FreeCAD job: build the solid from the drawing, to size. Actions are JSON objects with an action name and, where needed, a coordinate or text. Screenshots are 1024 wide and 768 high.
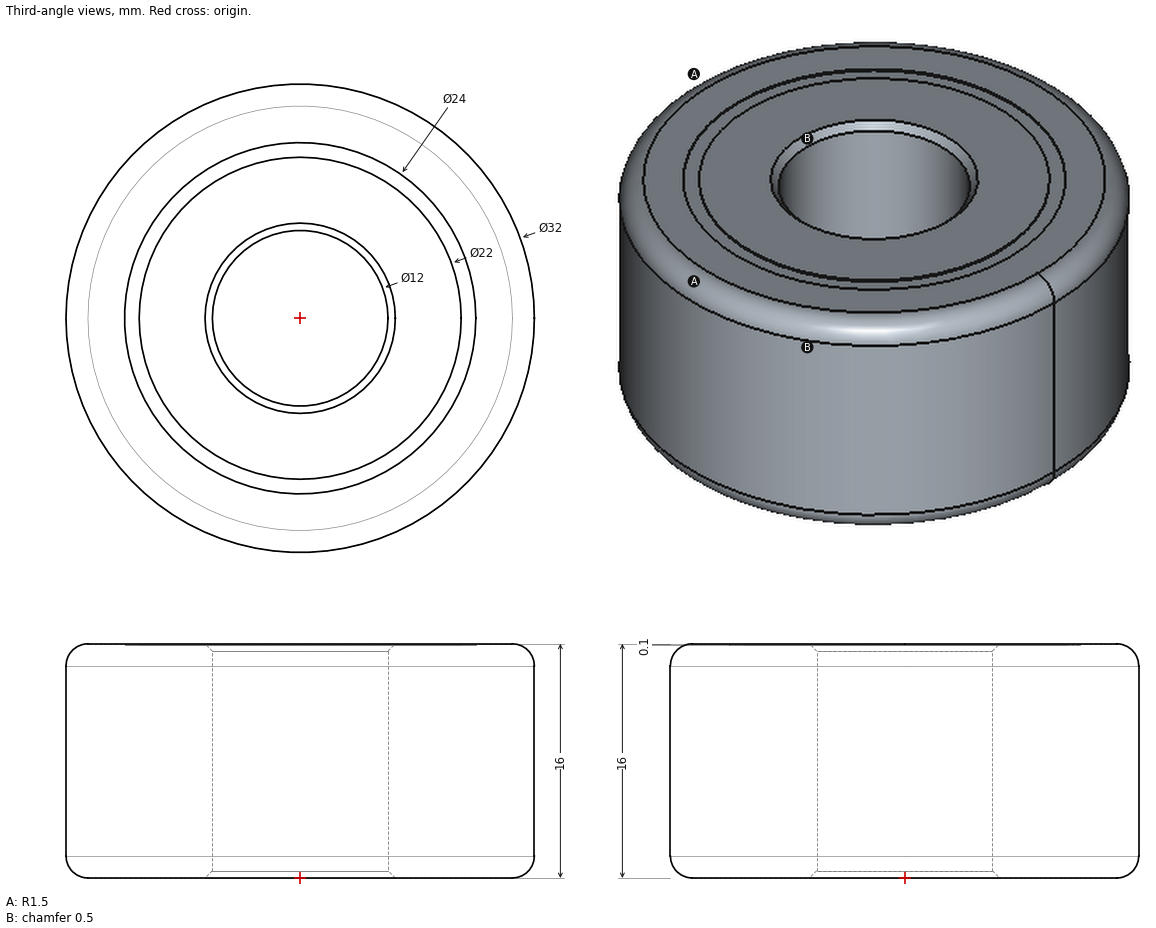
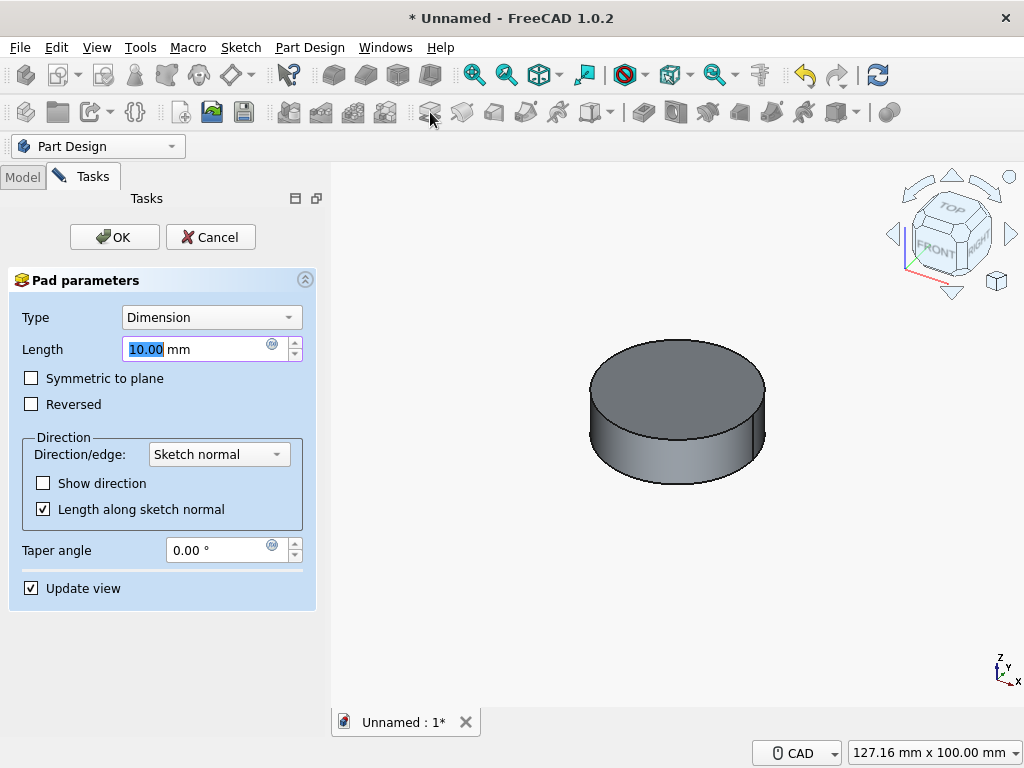
{"action": "type", "text": "16"}
{"action": "key", "text": "Tab"}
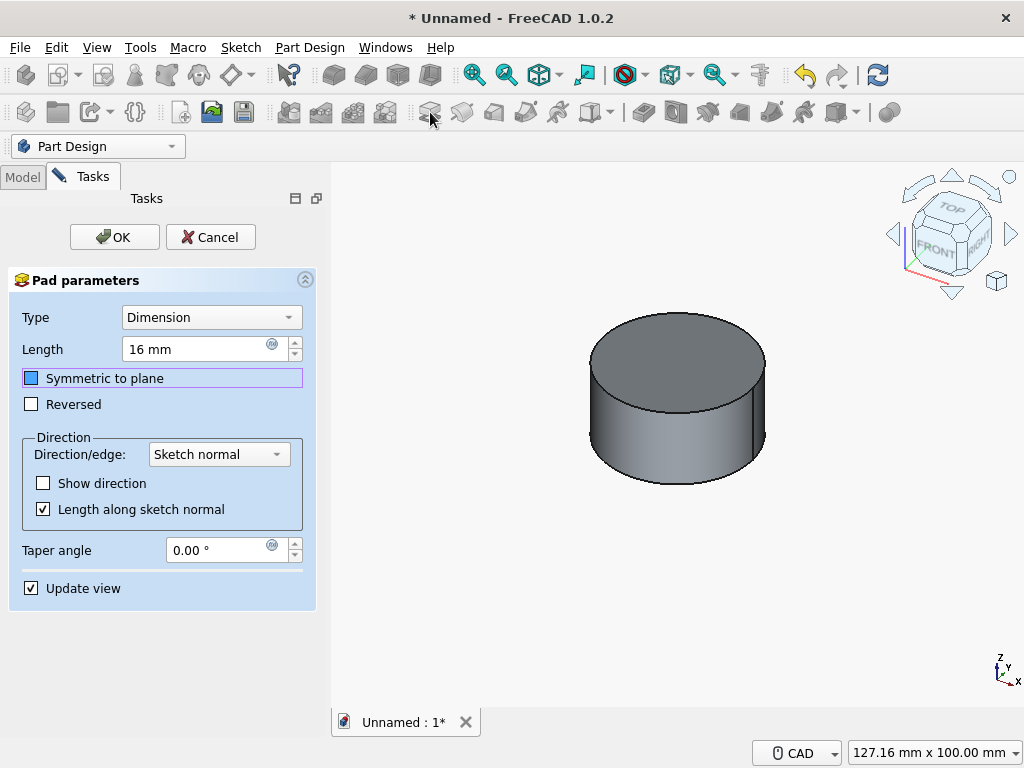
{"action": "left_click", "coordinate": [115, 237]}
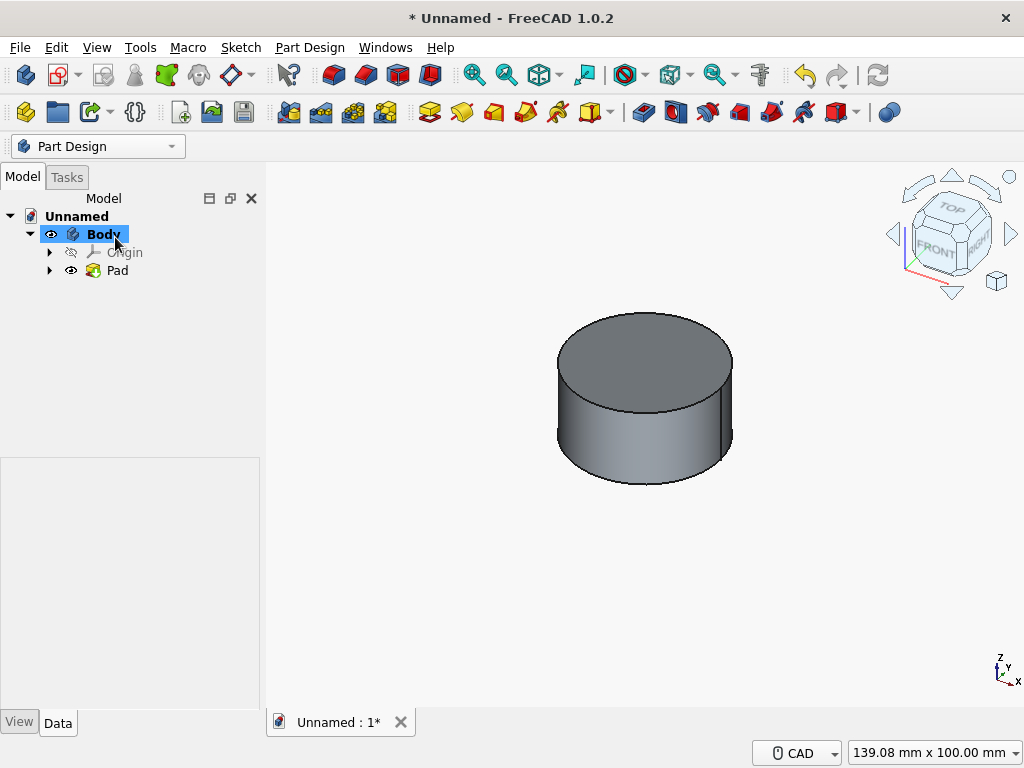
{"action": "left_click", "coordinate": [476, 76]}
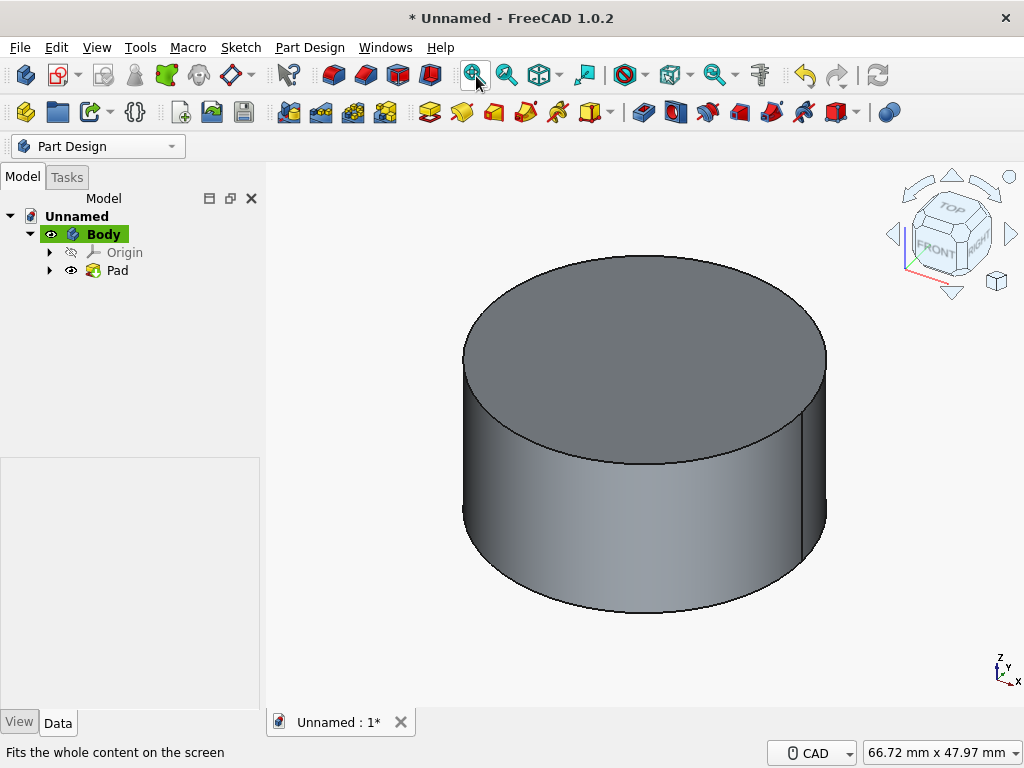
{"action": "left_click", "coordinate": [645, 359]}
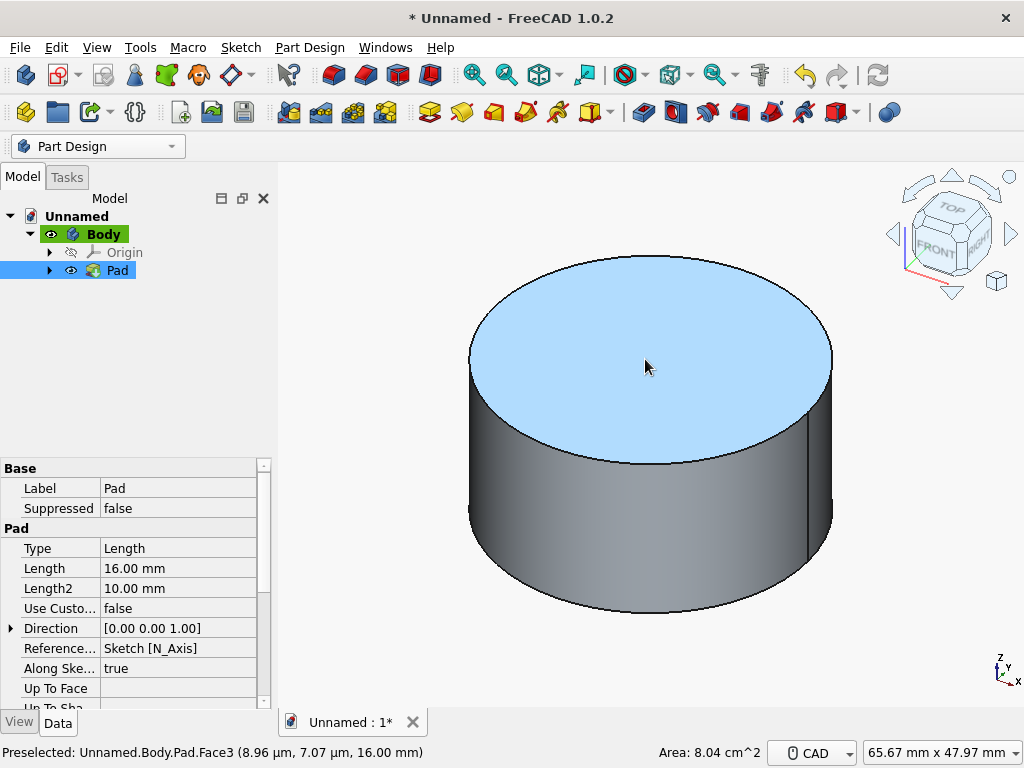
{"action": "left_click", "coordinate": [58, 76]}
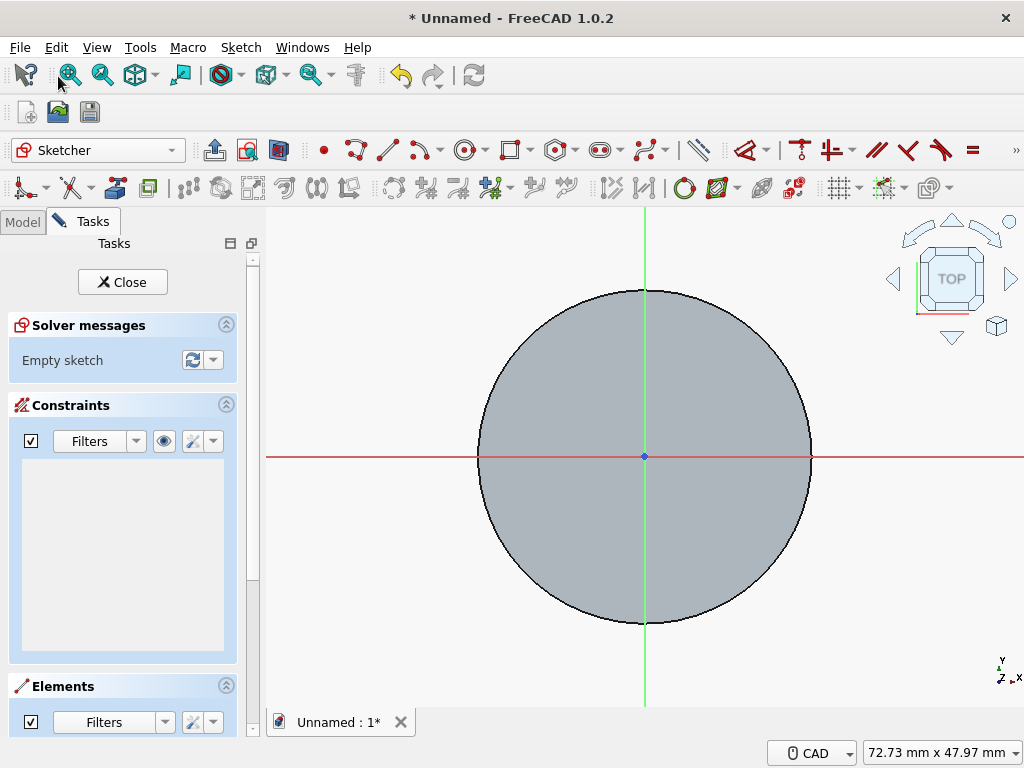
{"action": "scroll", "coordinate": [685, 457], "scroll_direction": "up", "scroll_amount": 5}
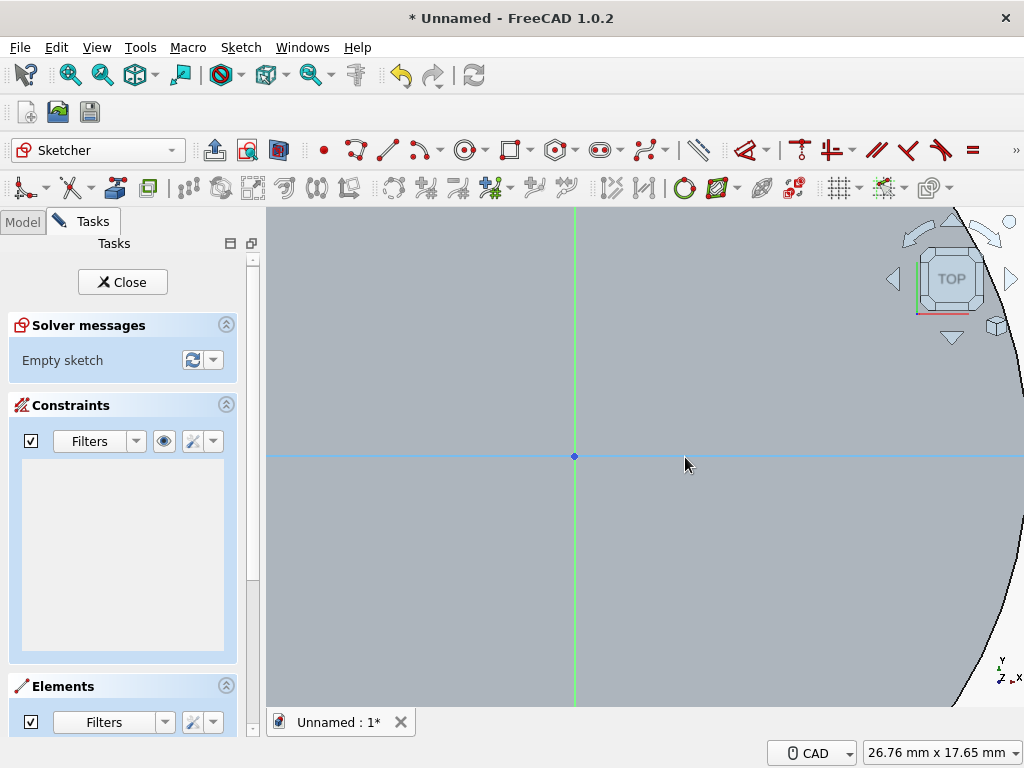
{"action": "left_click", "coordinate": [466, 150]}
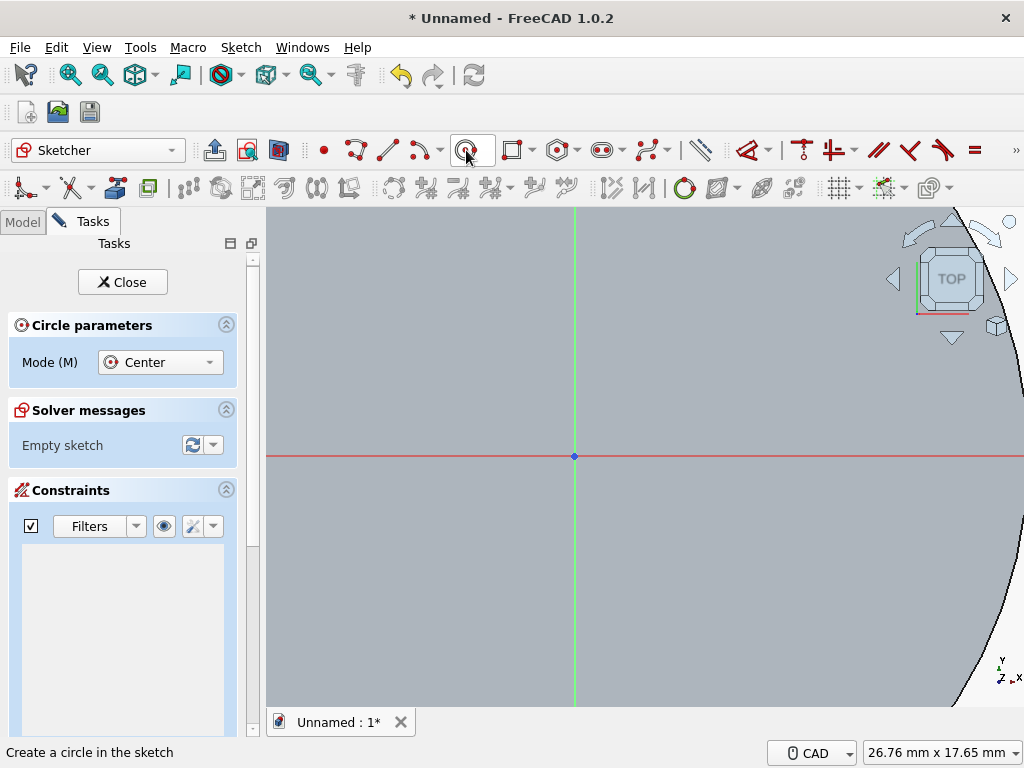
{"action": "left_click", "coordinate": [575, 456]}
{"action": "left_click", "coordinate": [695, 336]}
{"action": "key", "text": "Escape"}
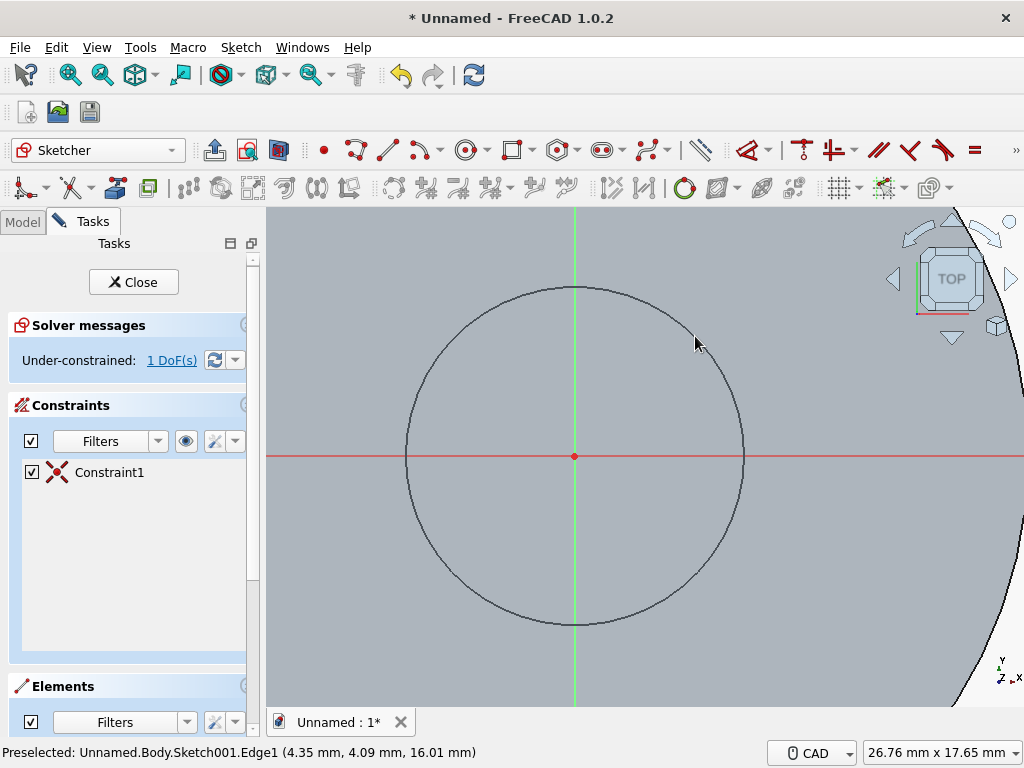
{"action": "left_click", "coordinate": [694, 336]}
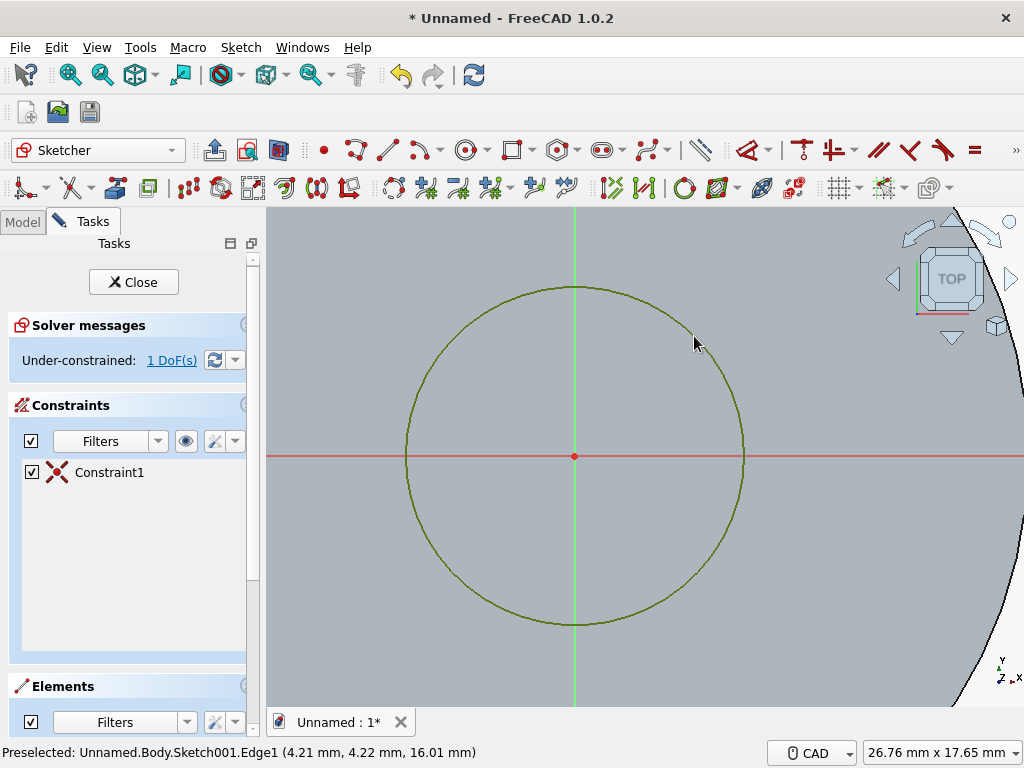
{"action": "left_click", "coordinate": [770, 150]}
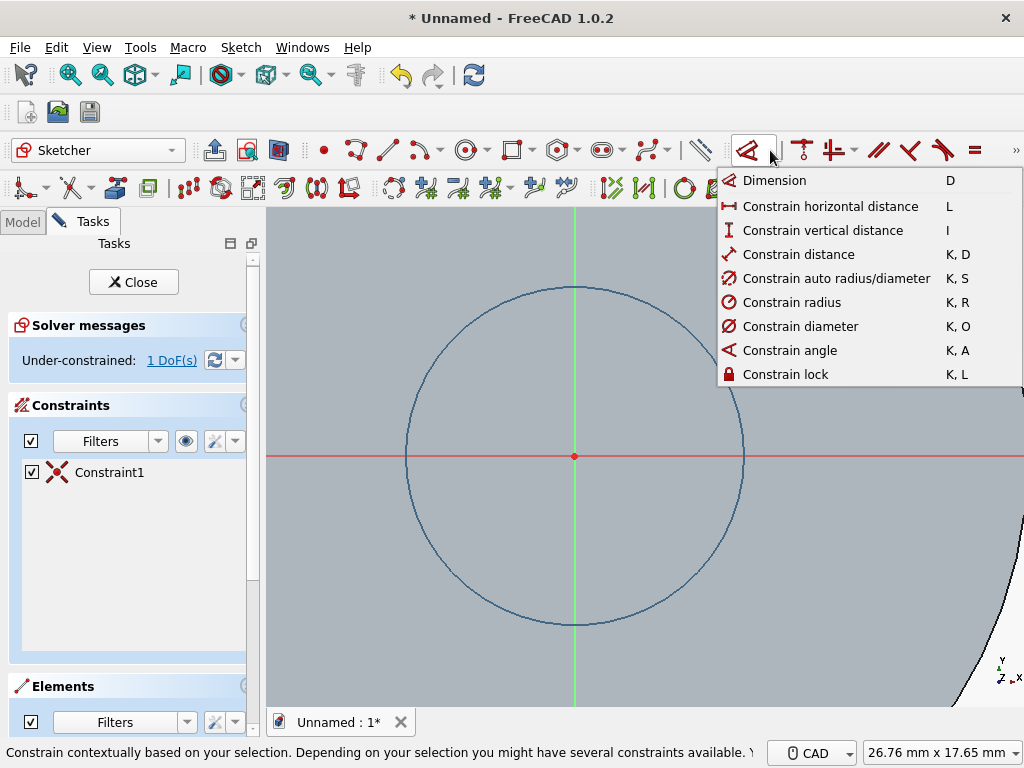
{"action": "left_click", "coordinate": [870, 326]}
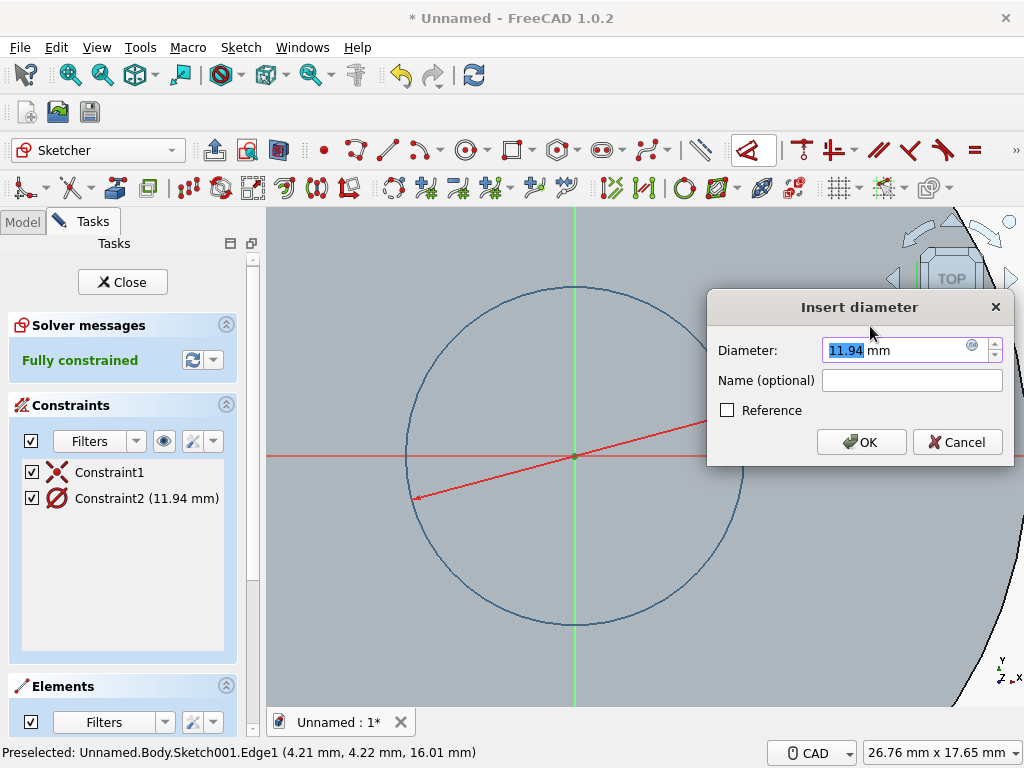
{"action": "type", "text": "12"}
{"action": "key", "text": "Return"}